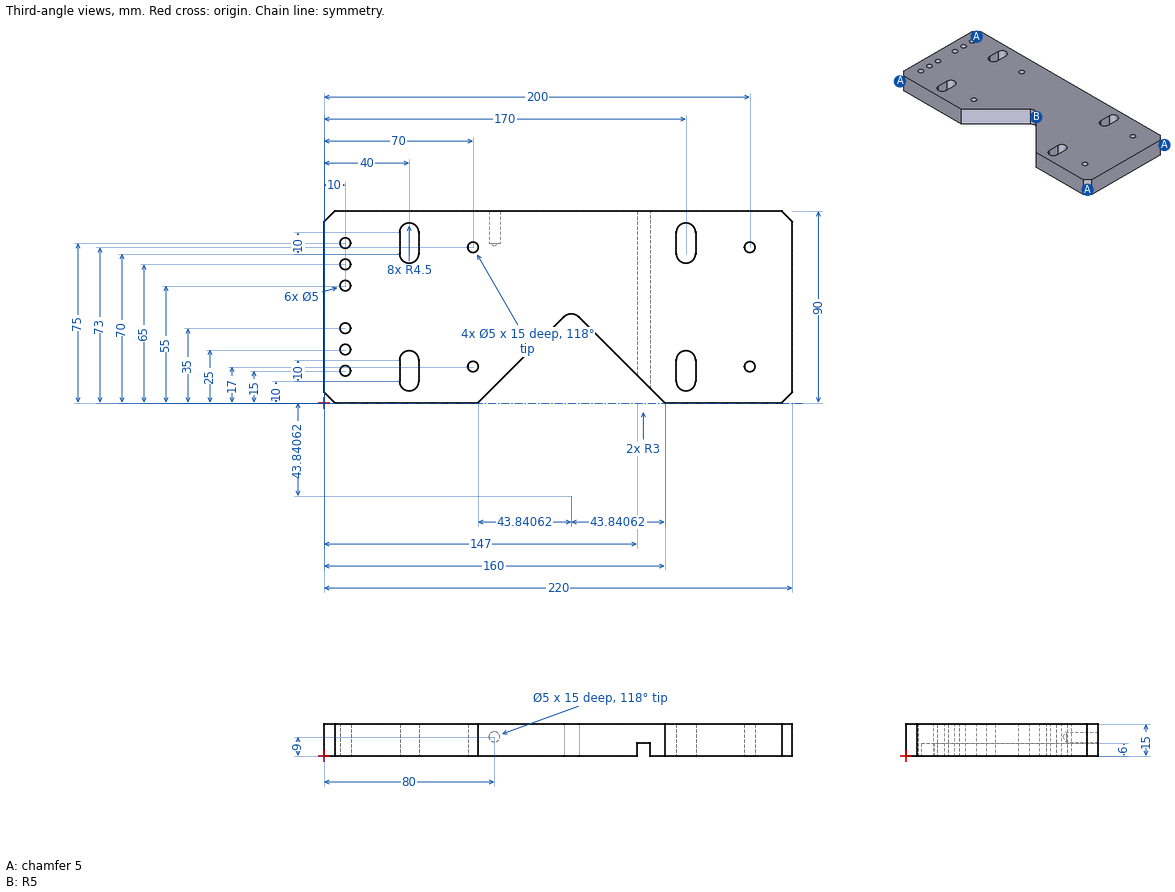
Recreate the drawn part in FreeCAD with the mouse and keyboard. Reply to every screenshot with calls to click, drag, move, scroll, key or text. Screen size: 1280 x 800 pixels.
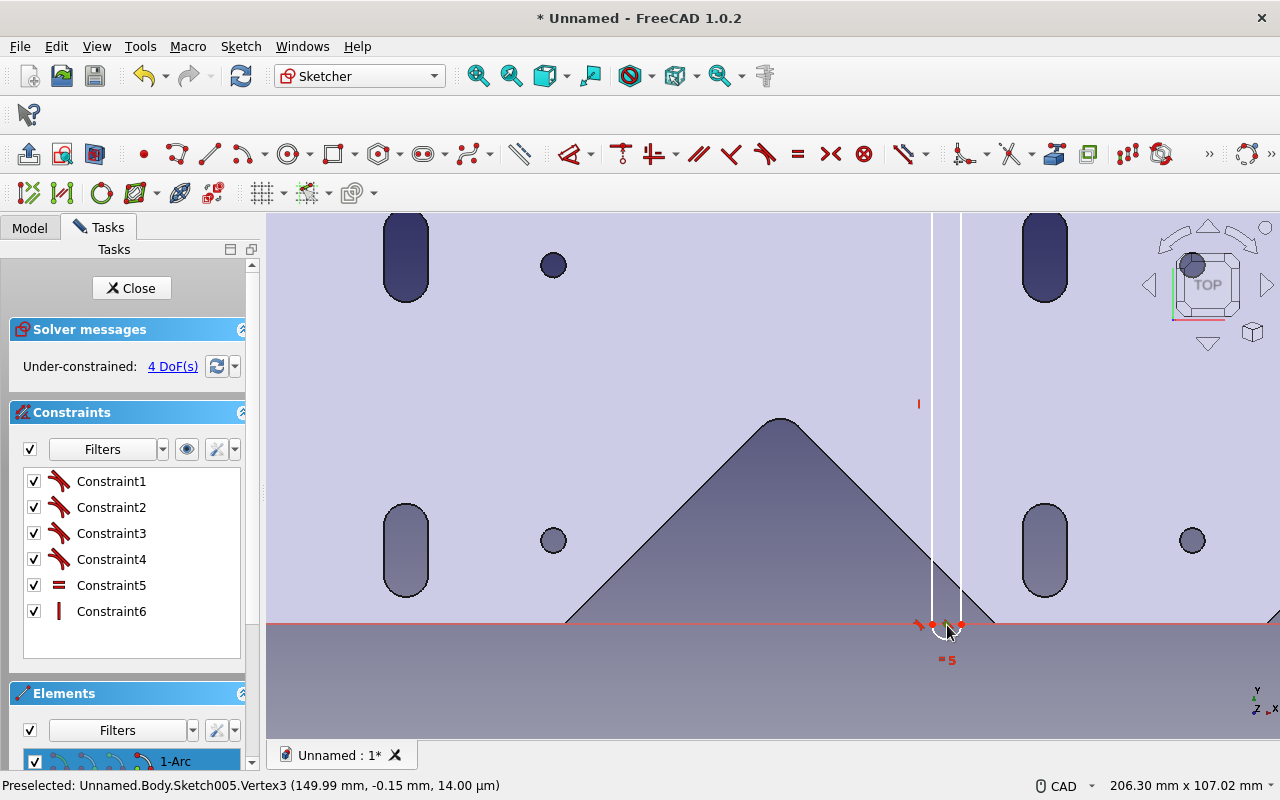
click(353, 624)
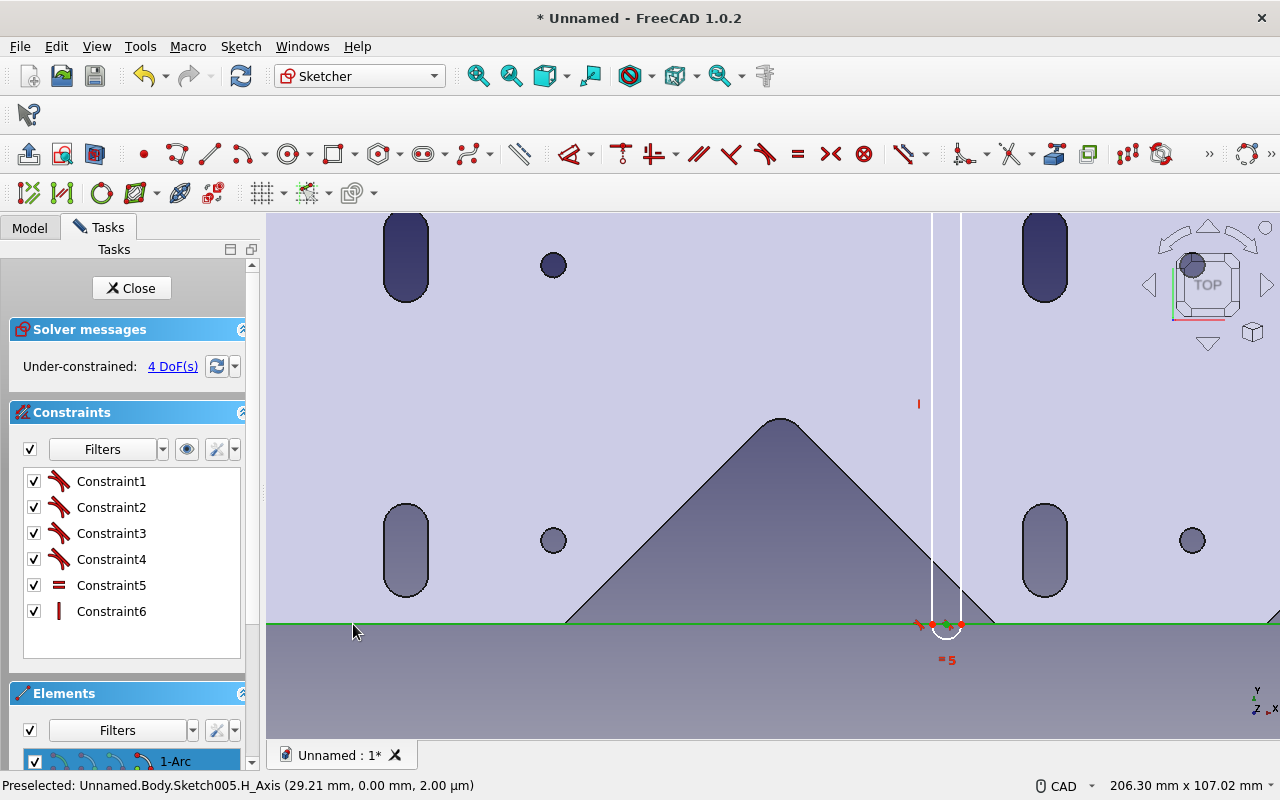
key(c)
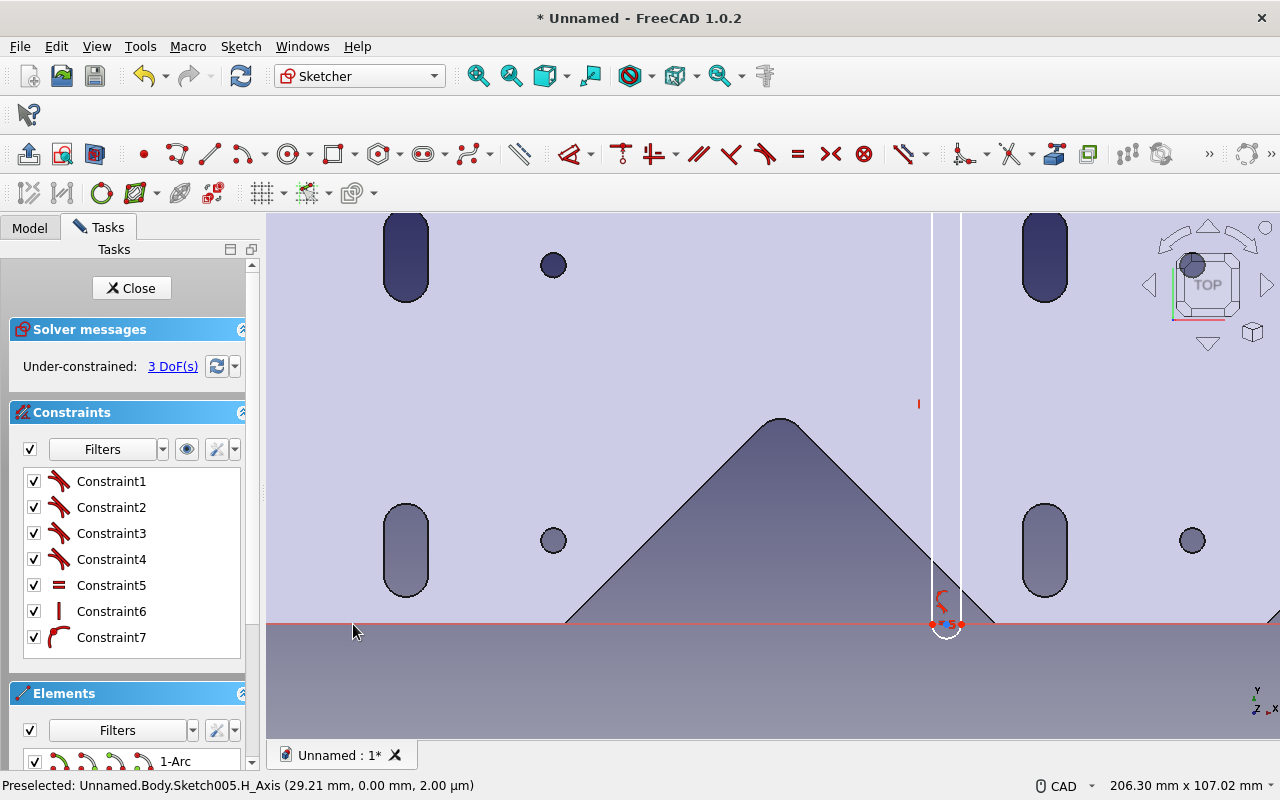
key(d)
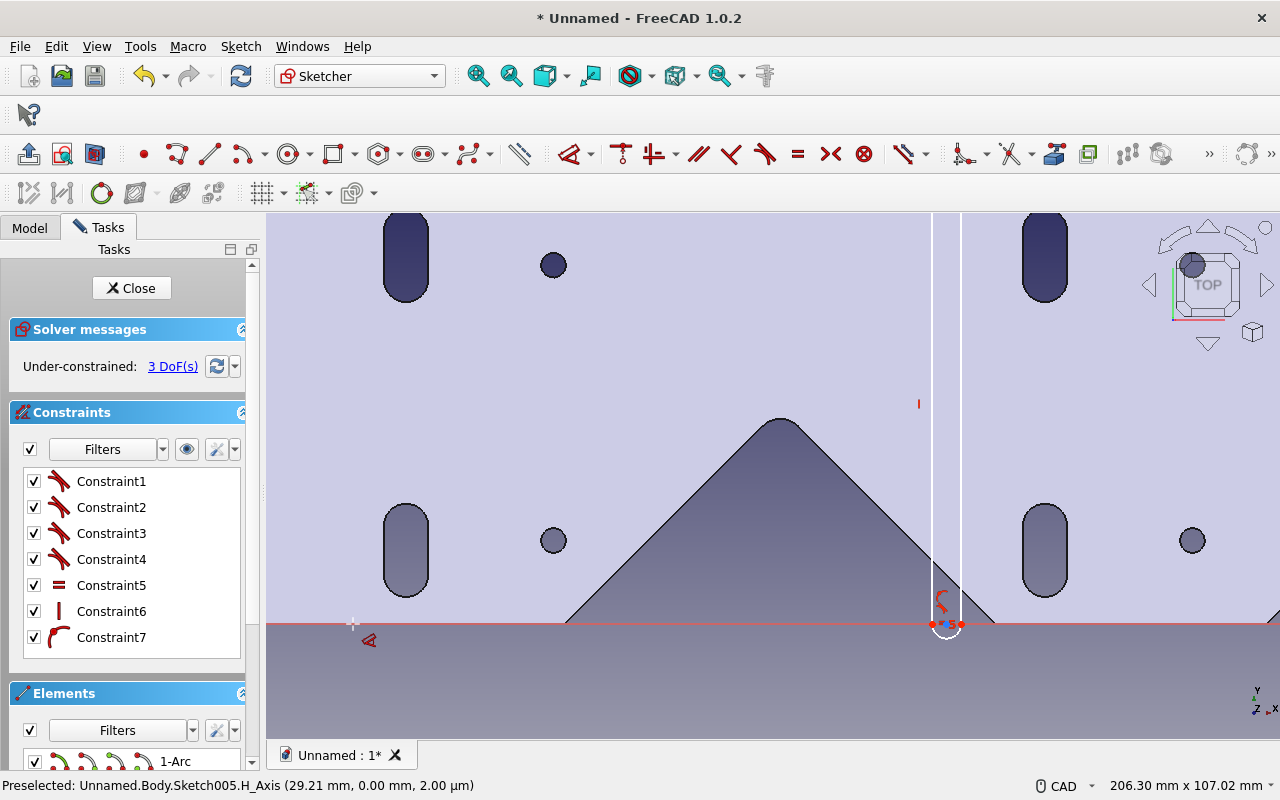
scroll(938, 636, up, 5)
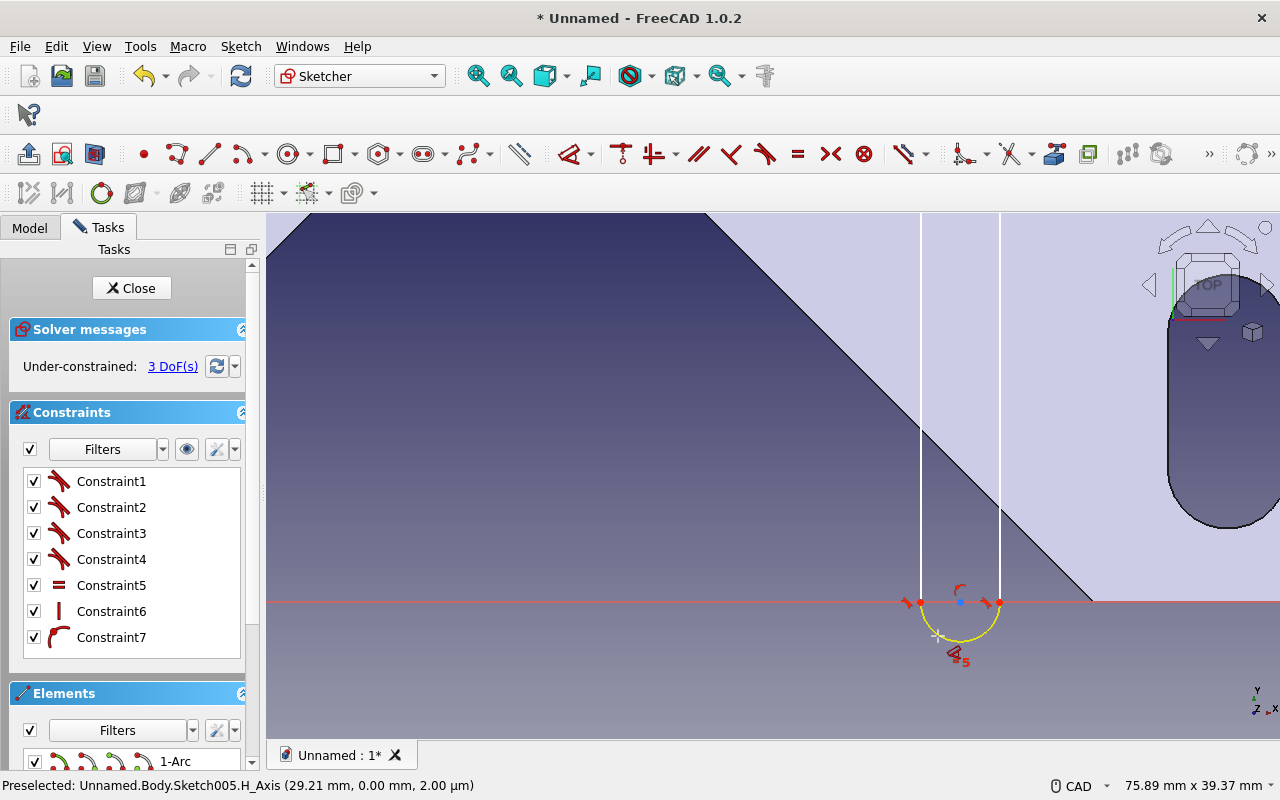
click(937, 634)
click(918, 660)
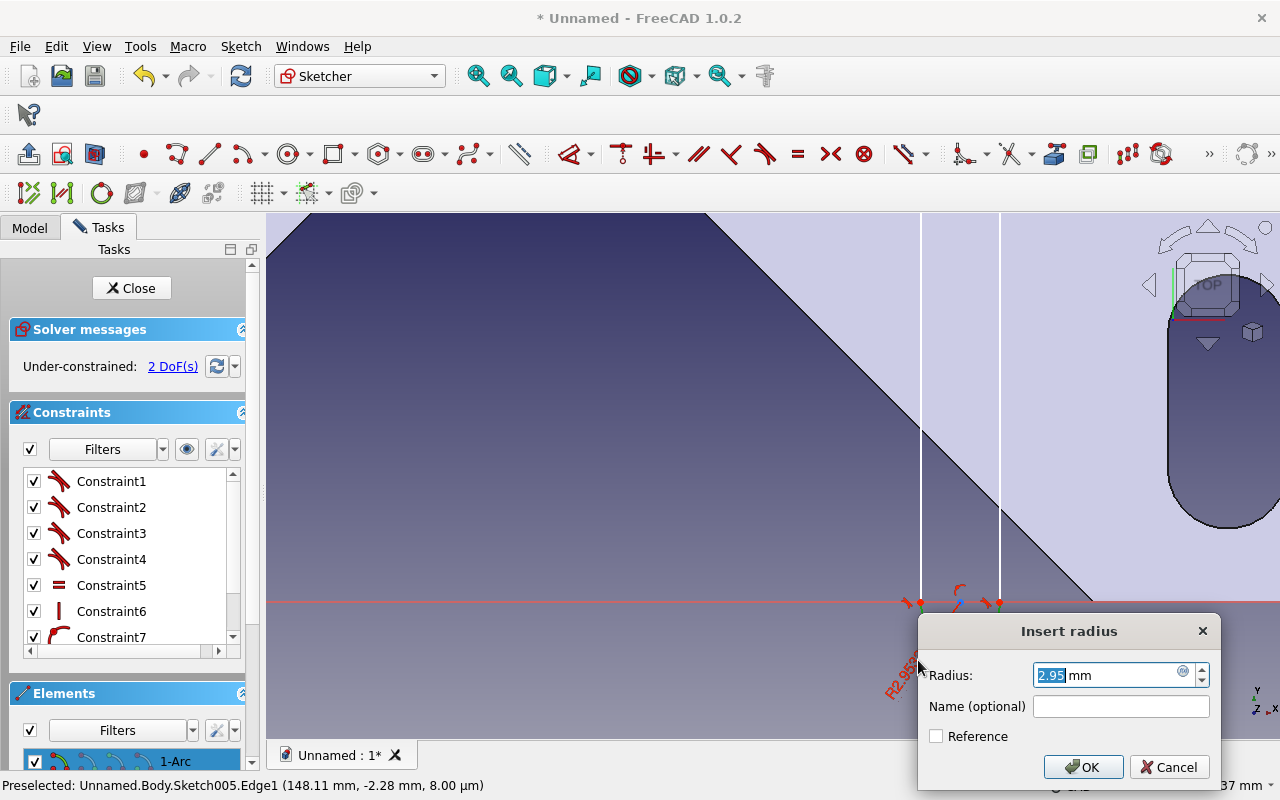
text(3)
key(Return)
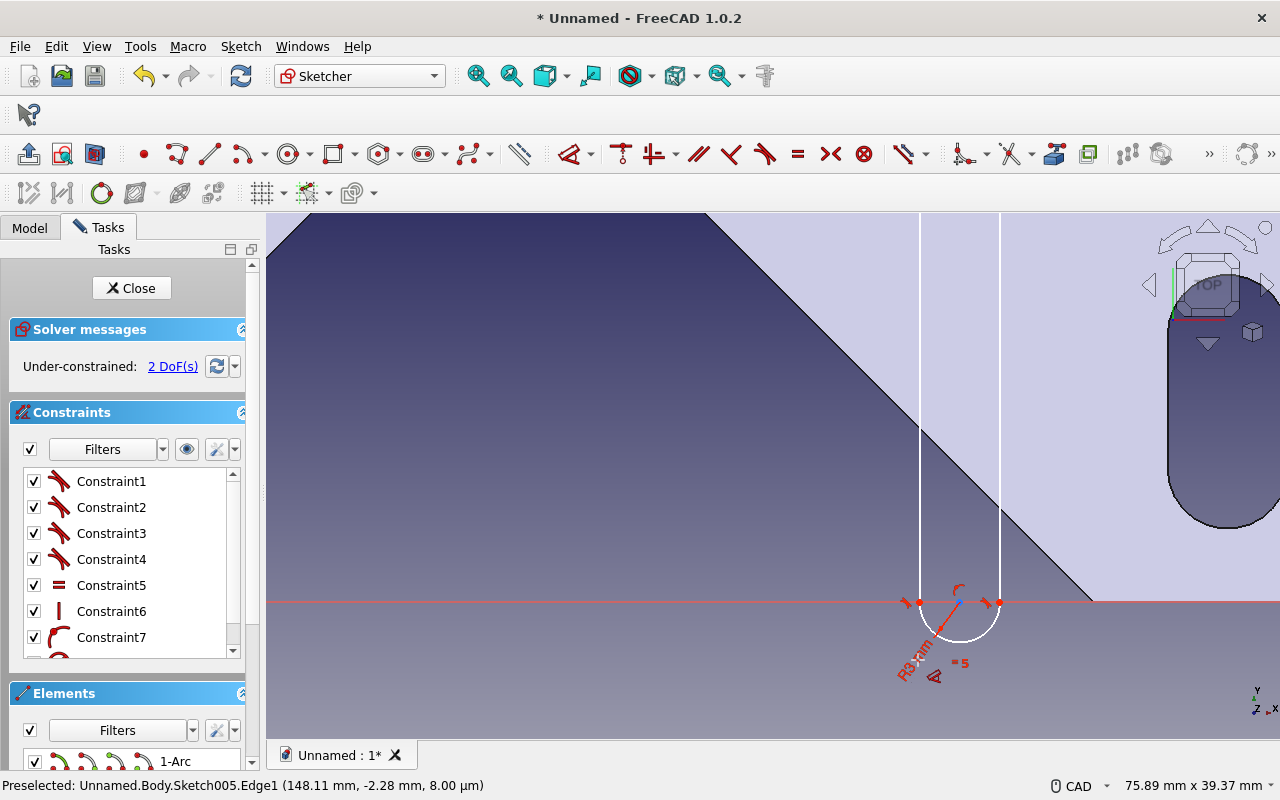
scroll(942, 631, down, 7)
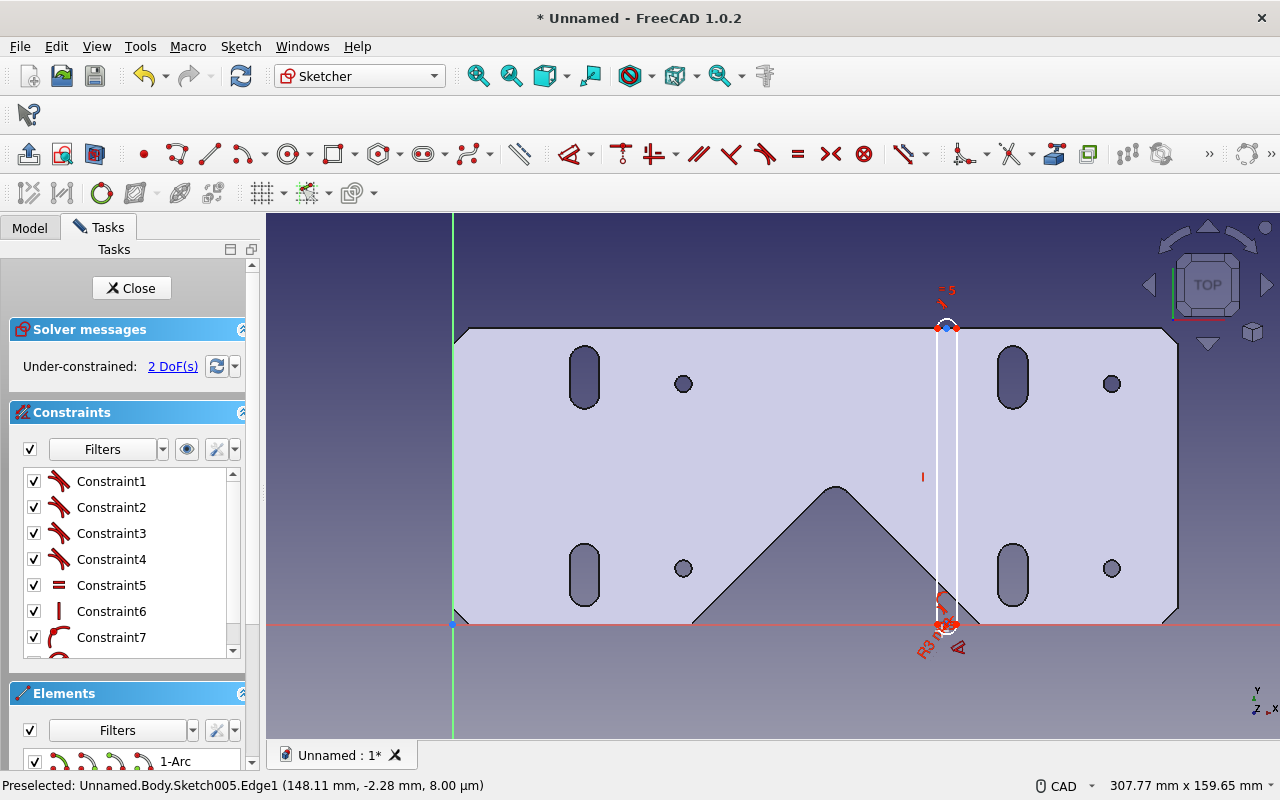
click(937, 536)
click(971, 477)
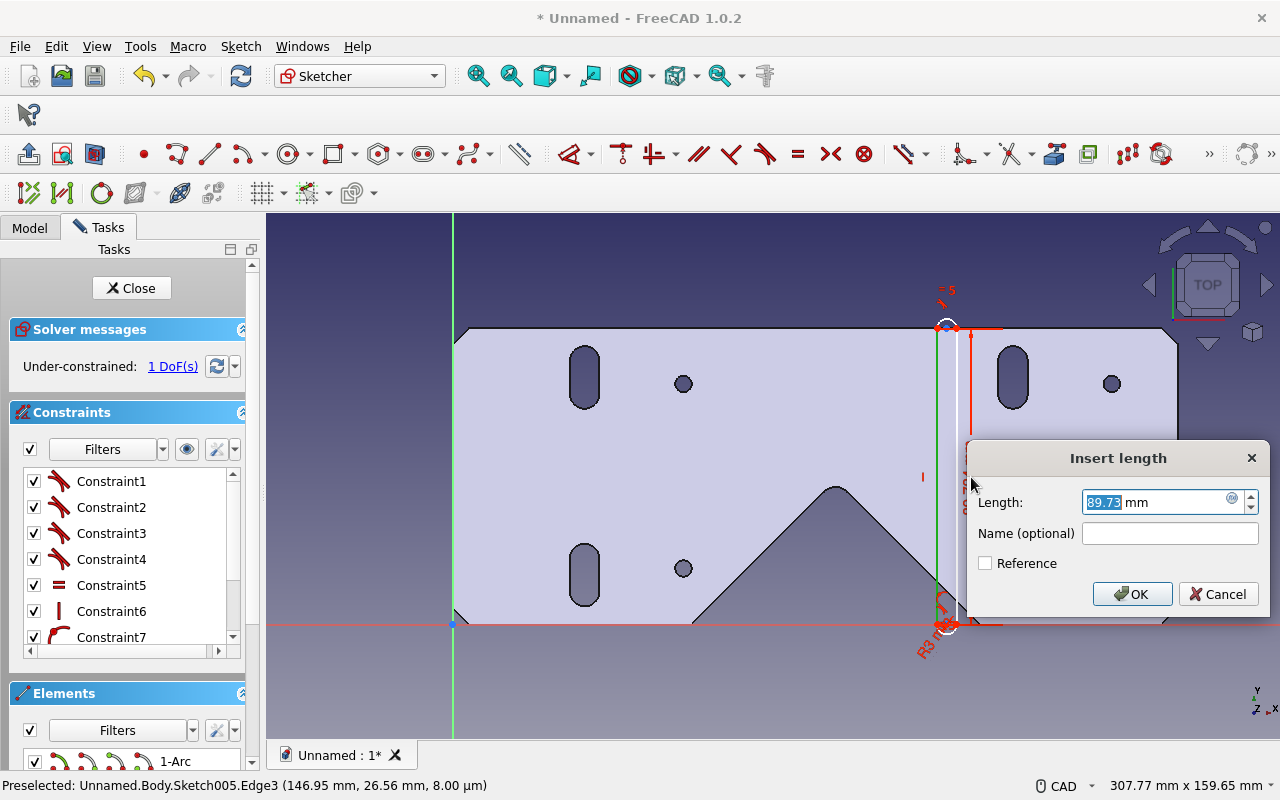
text(90)
key(Return)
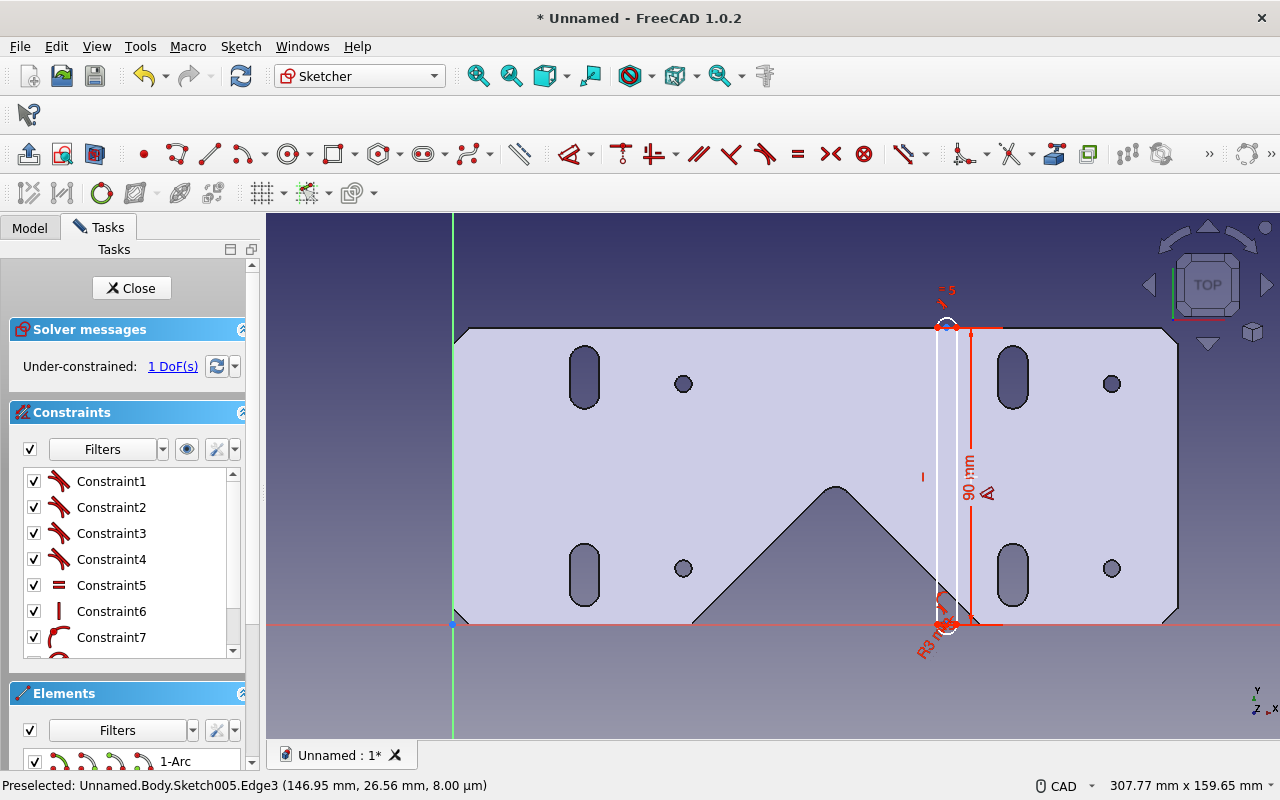
scroll(937, 625, up, 2)